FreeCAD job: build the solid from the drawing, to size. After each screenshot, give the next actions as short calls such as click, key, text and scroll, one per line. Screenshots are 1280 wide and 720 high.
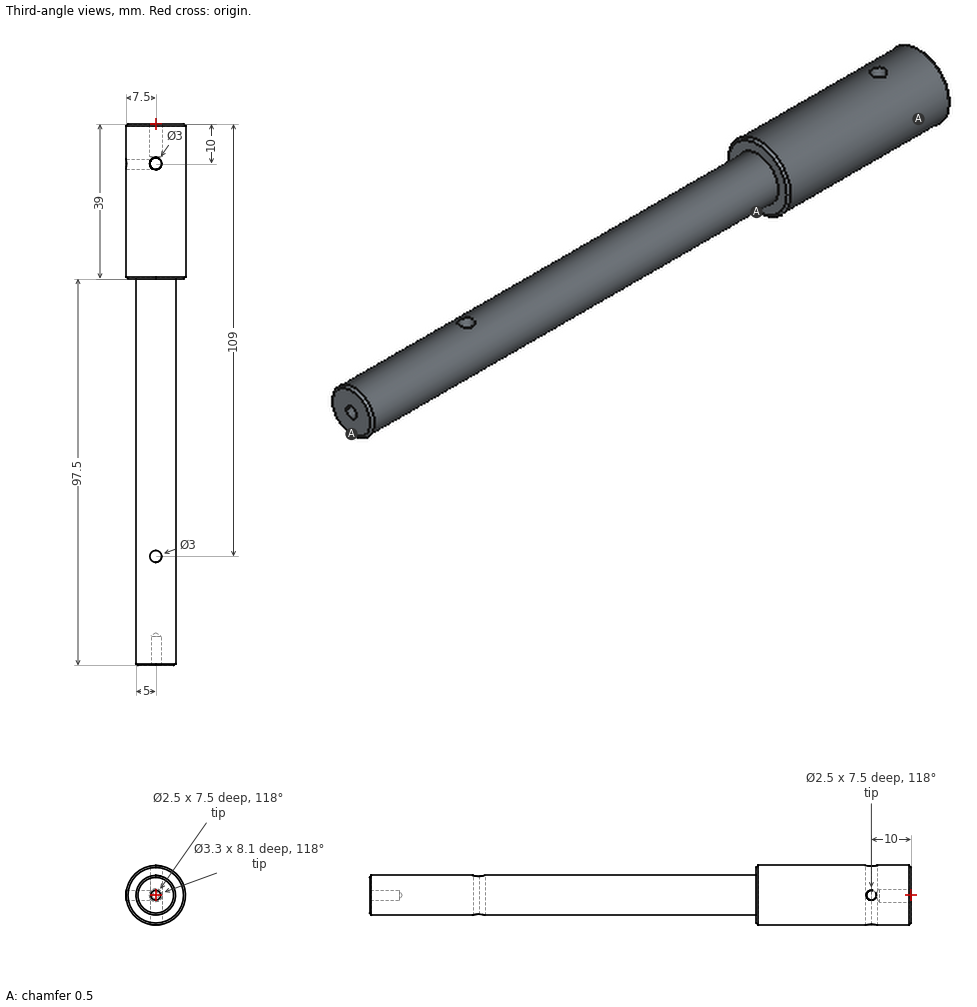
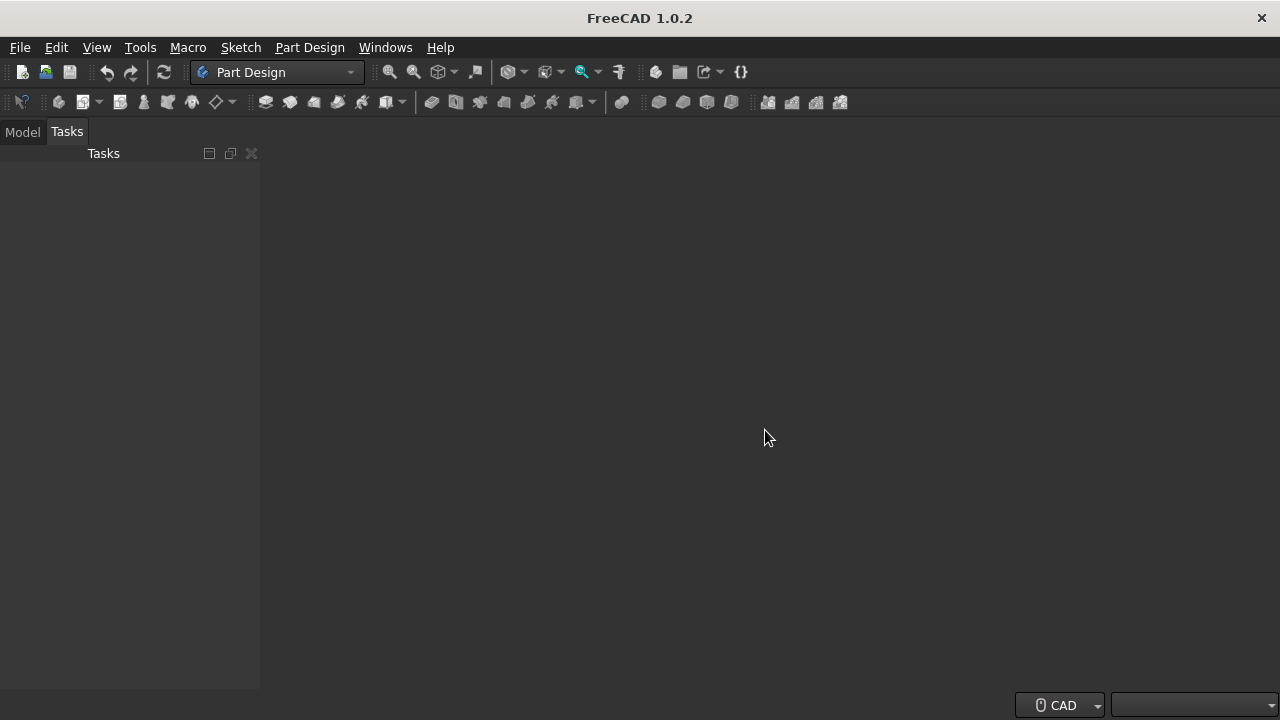
click(22, 72)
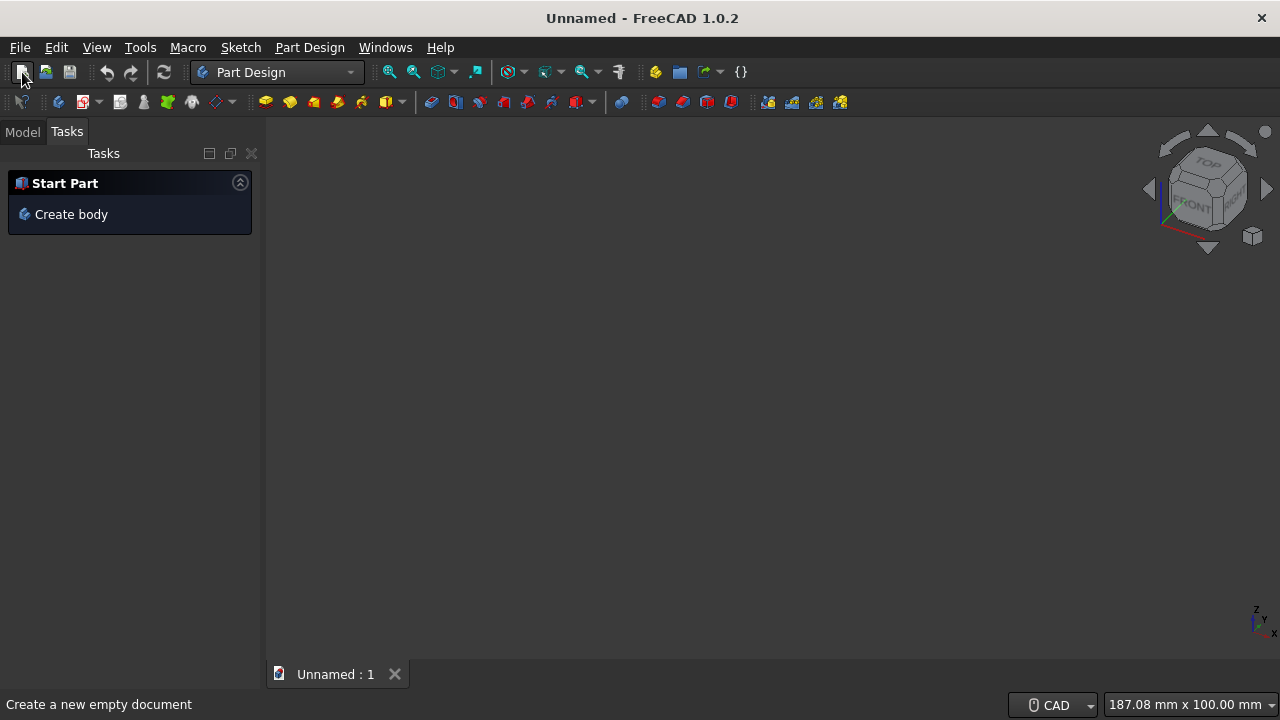
click(84, 102)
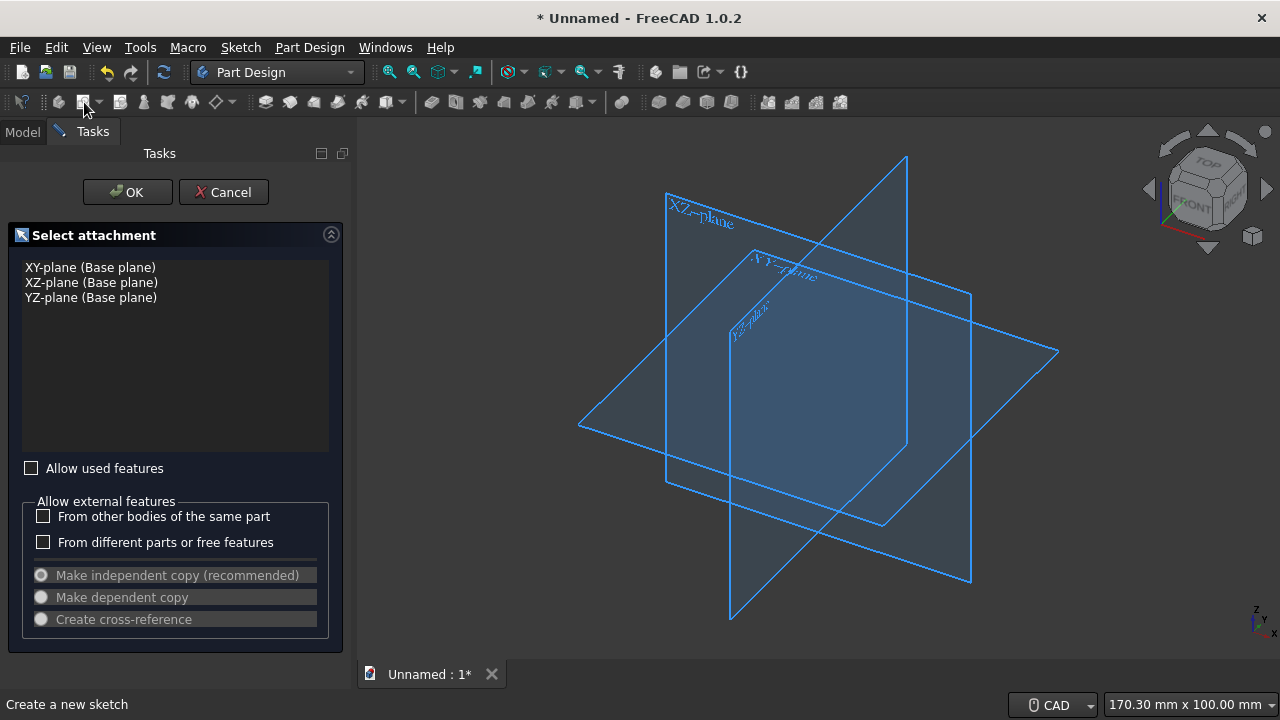
click(82, 268)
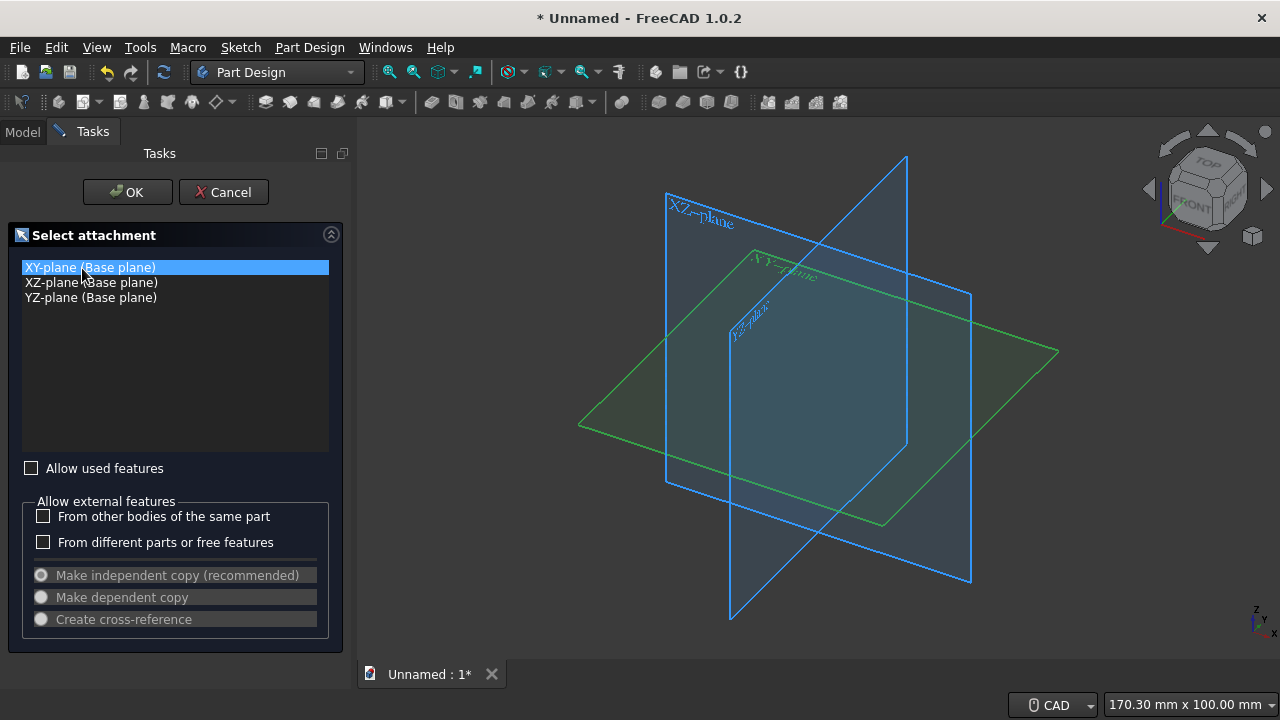
click(128, 192)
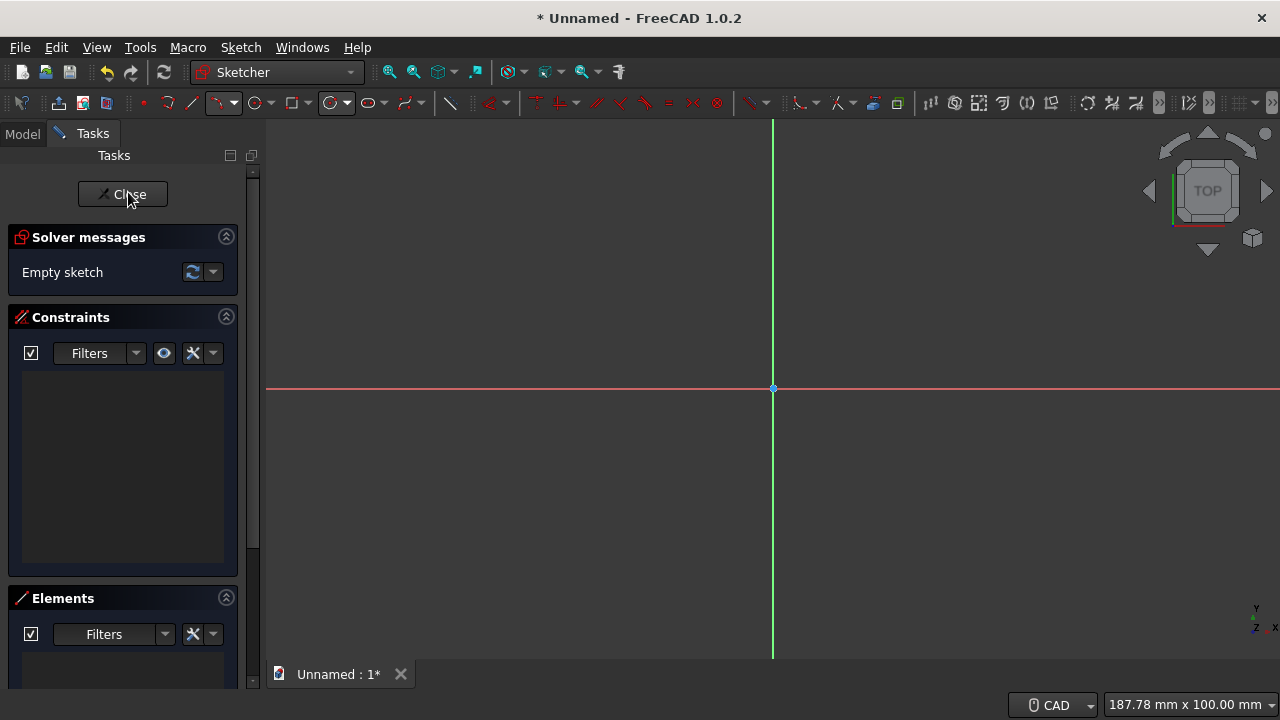
scroll(665, 147, down, 4)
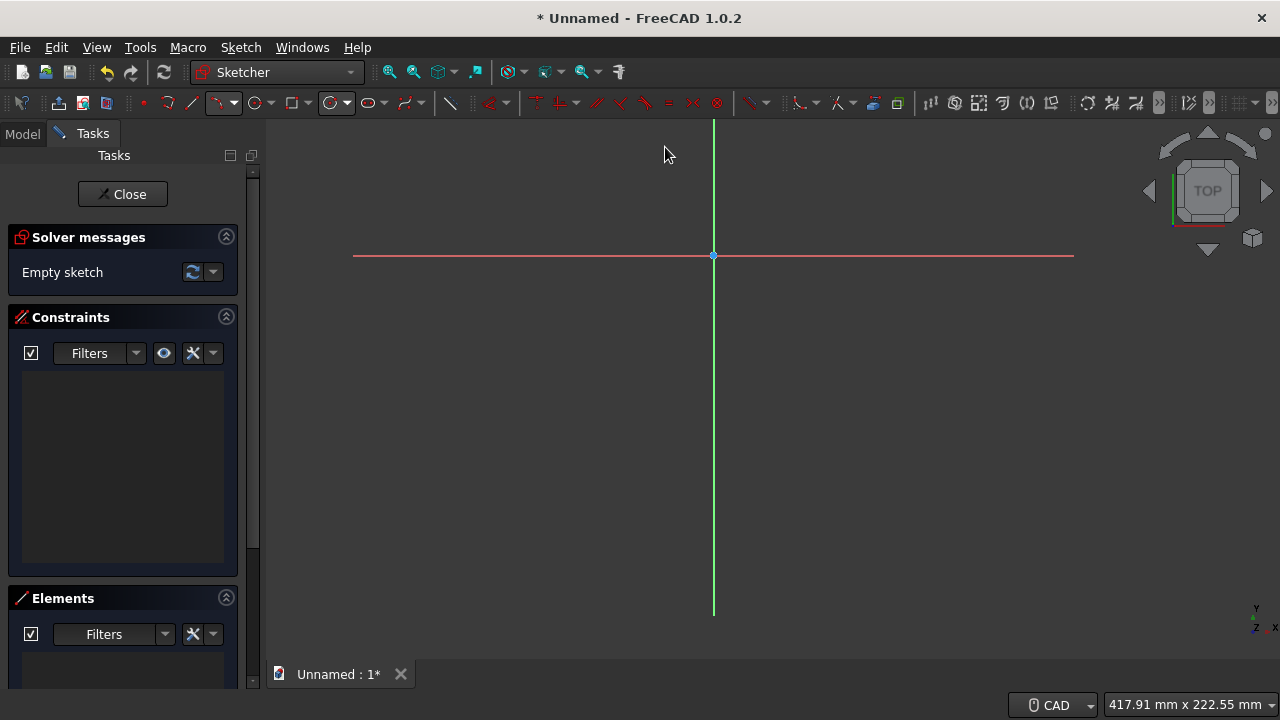
click(168, 104)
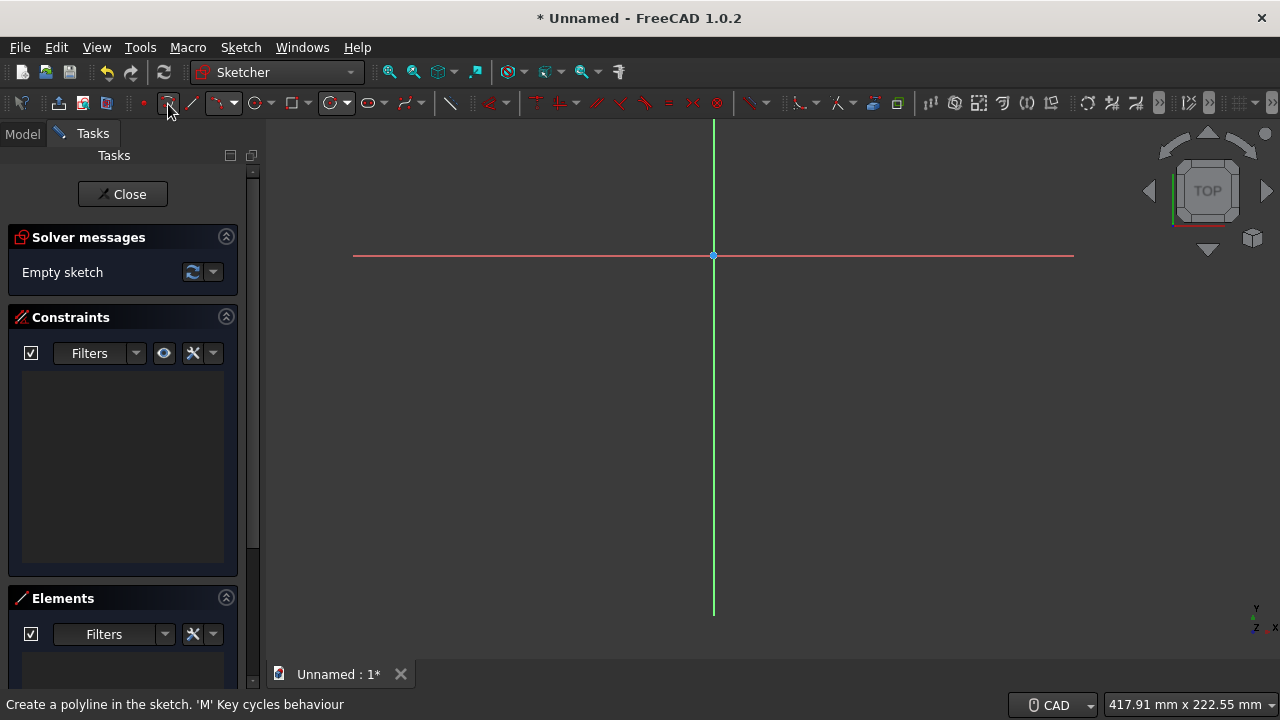
click(714, 256)
click(696, 265)
click(696, 350)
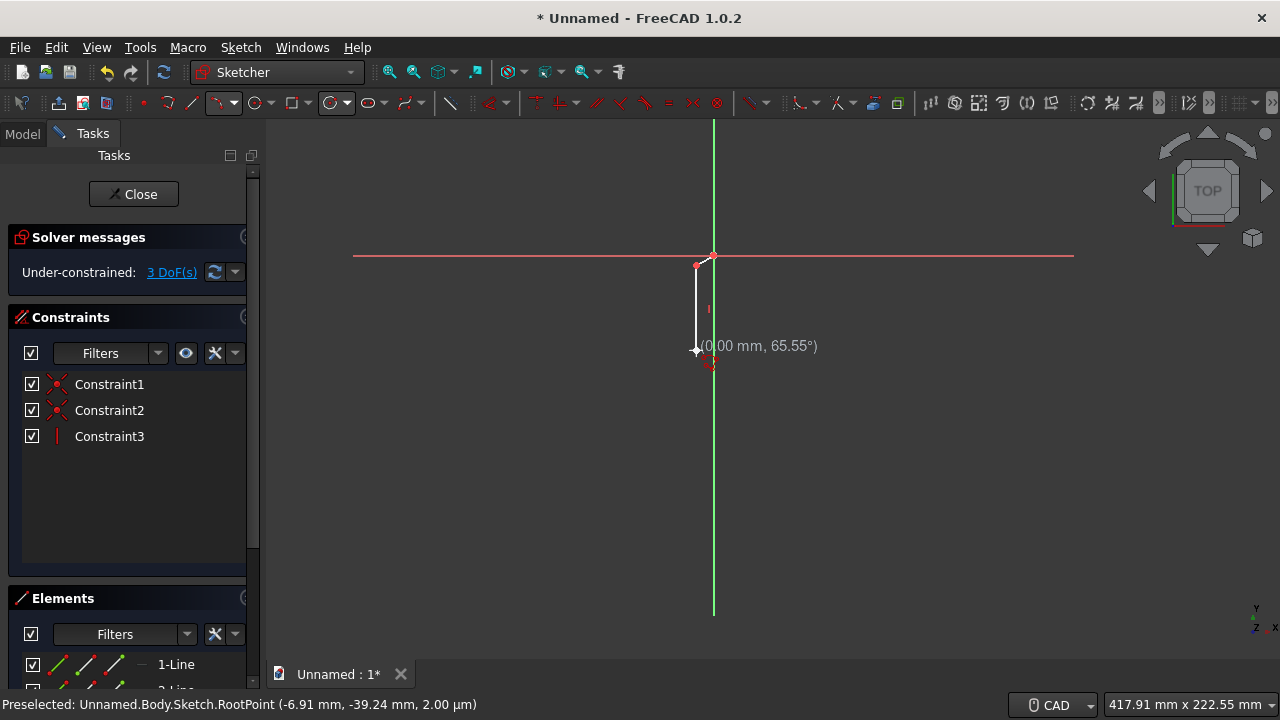
scroll(702, 350, up, 5)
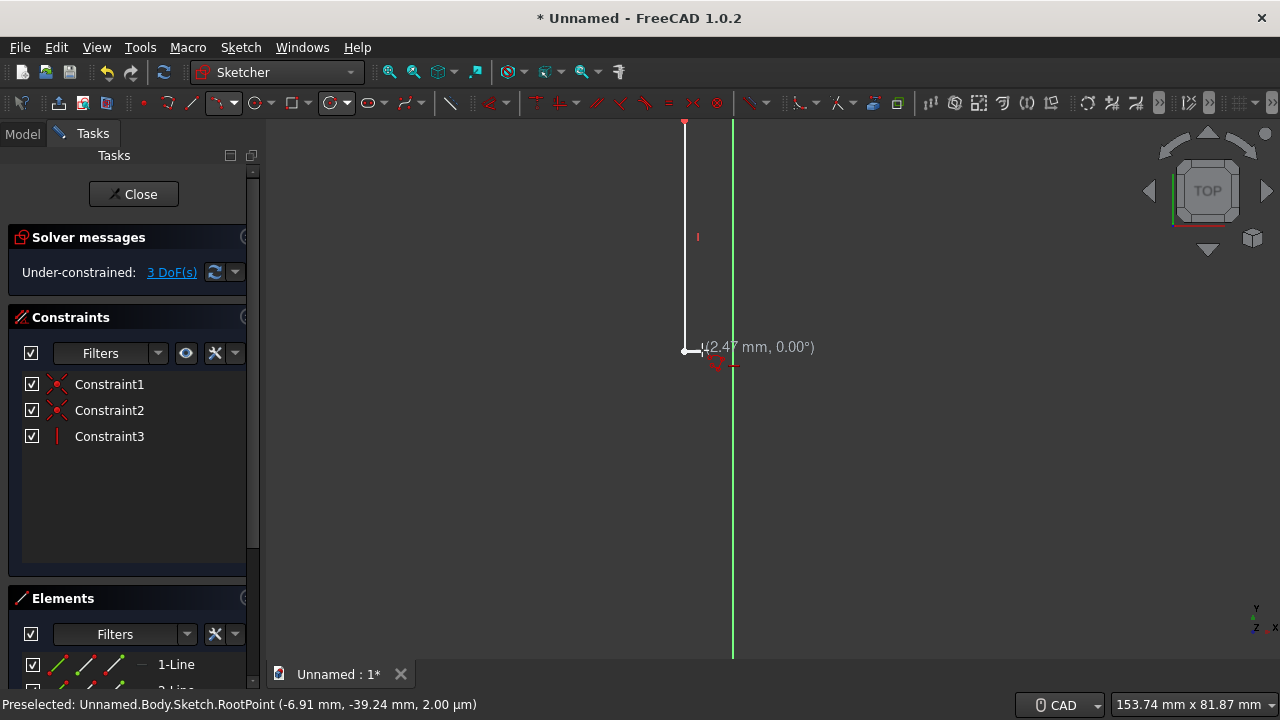
click(700, 349)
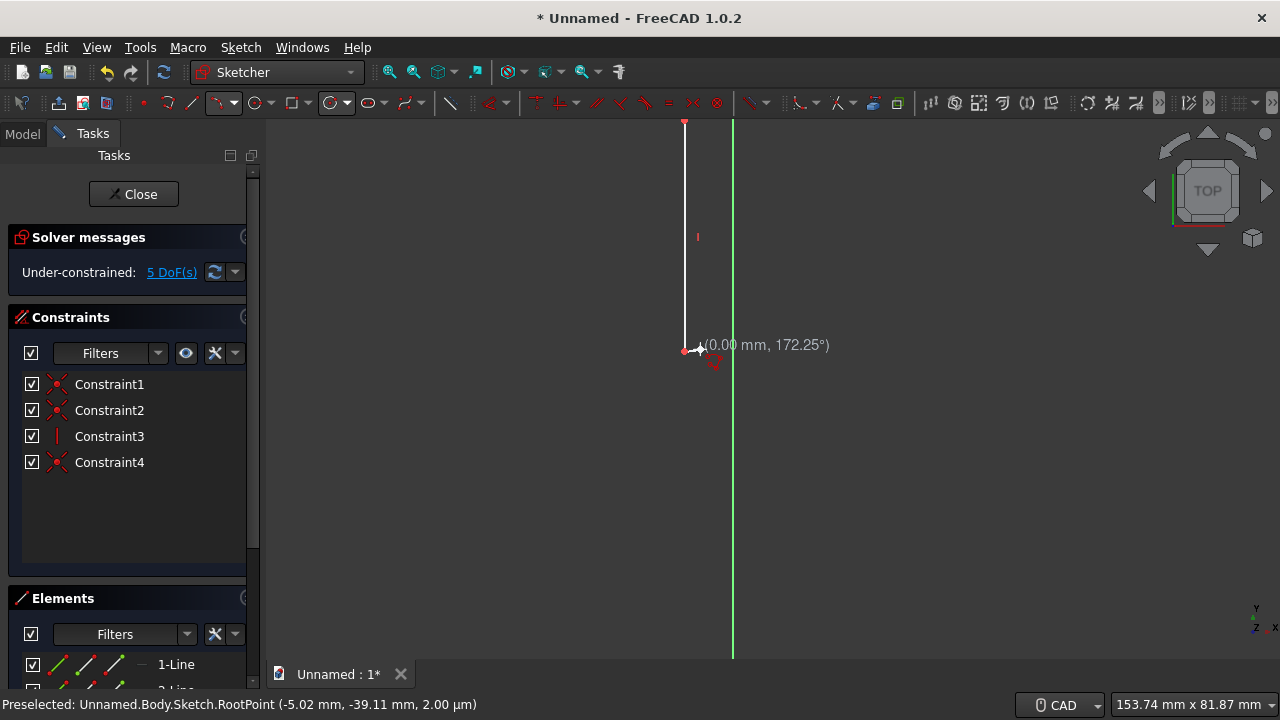
scroll(702, 299, down, 5)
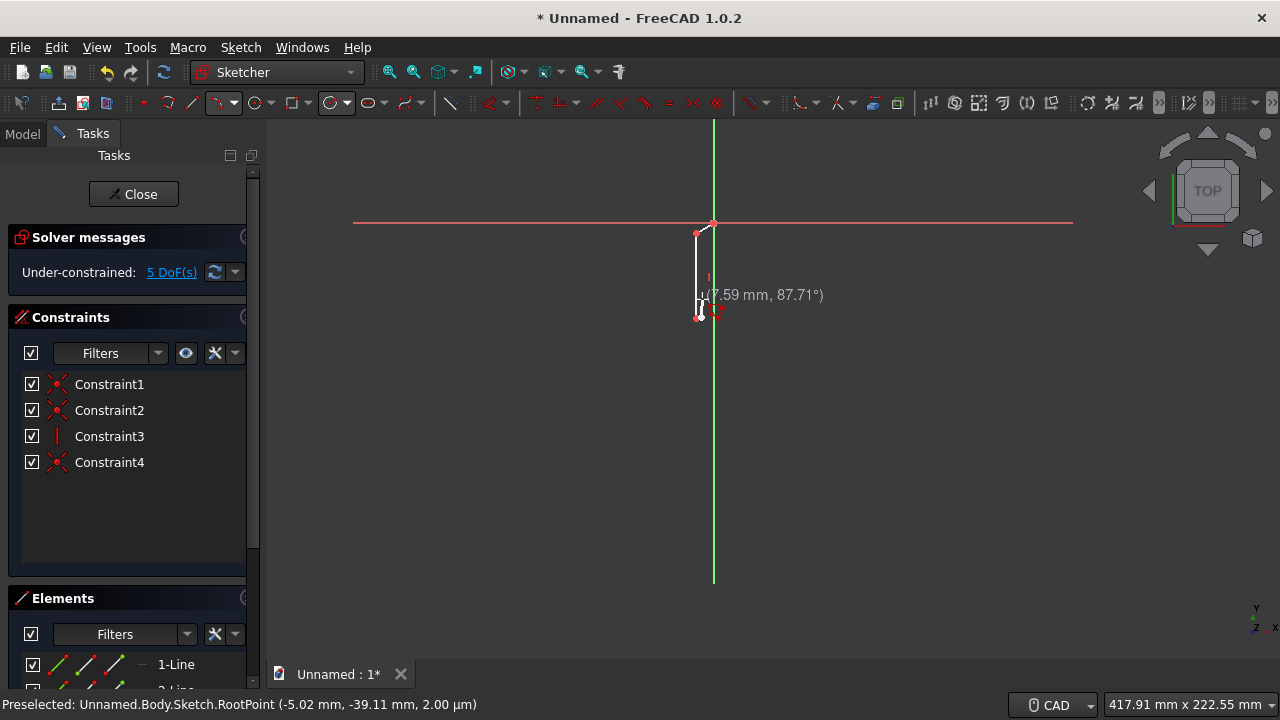
scroll(702, 555, up, 2)